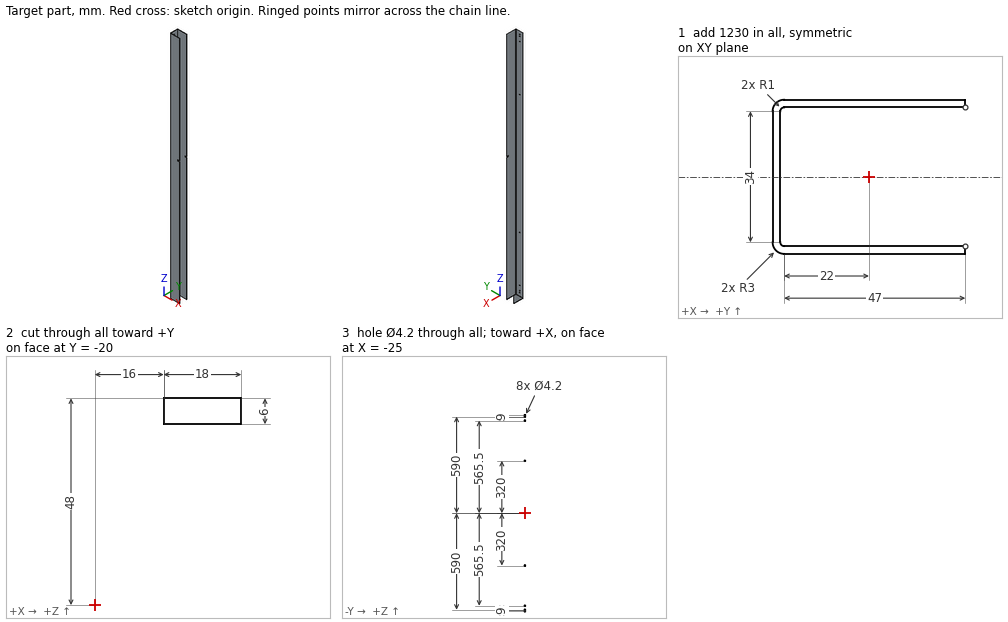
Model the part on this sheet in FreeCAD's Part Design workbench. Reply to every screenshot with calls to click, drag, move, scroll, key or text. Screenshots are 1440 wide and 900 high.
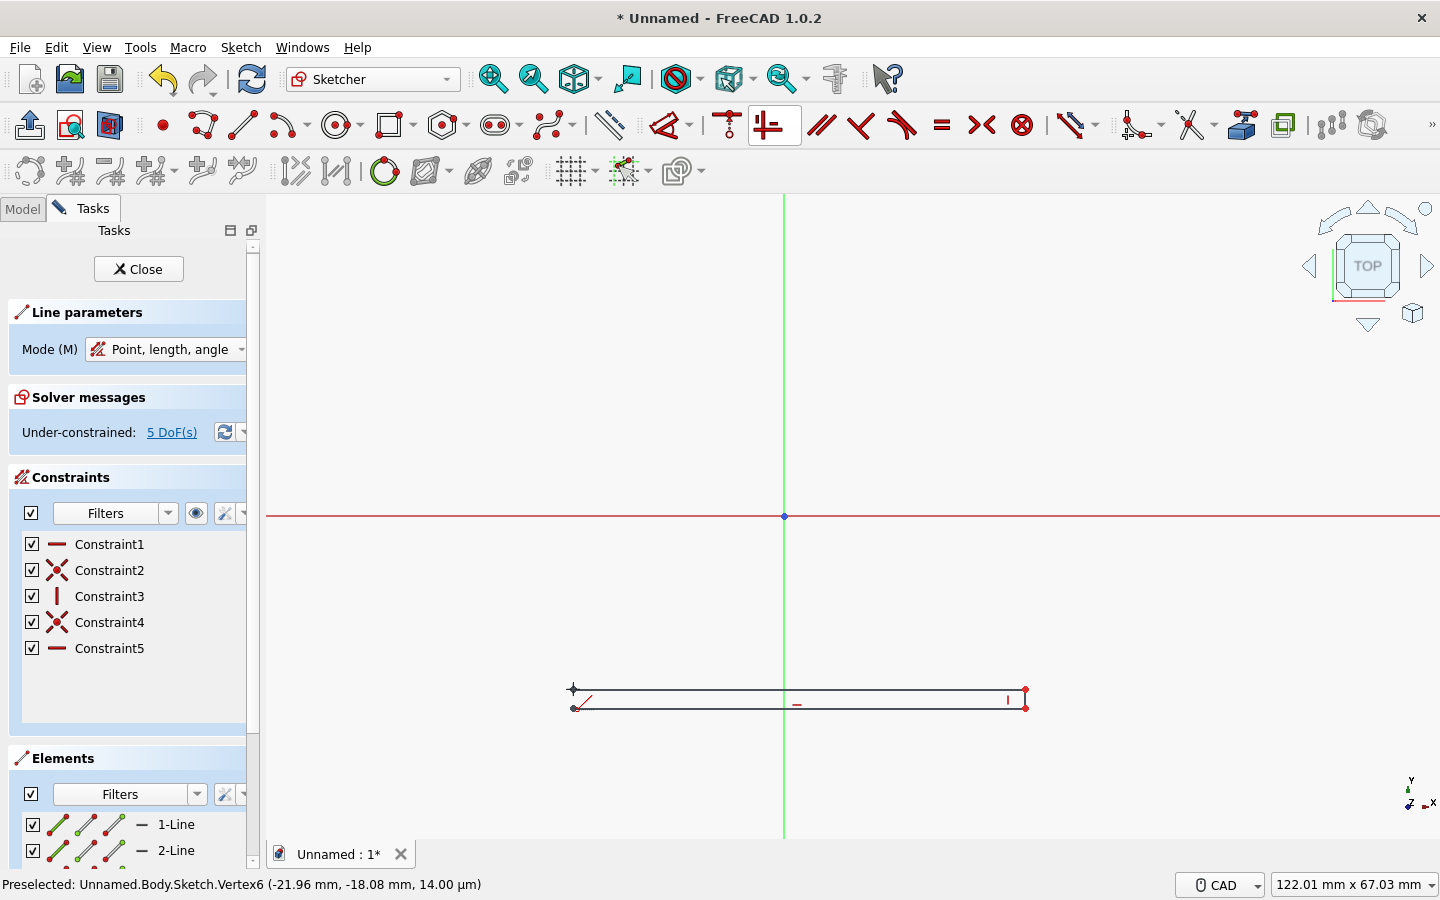
click(563, 680)
click(563, 352)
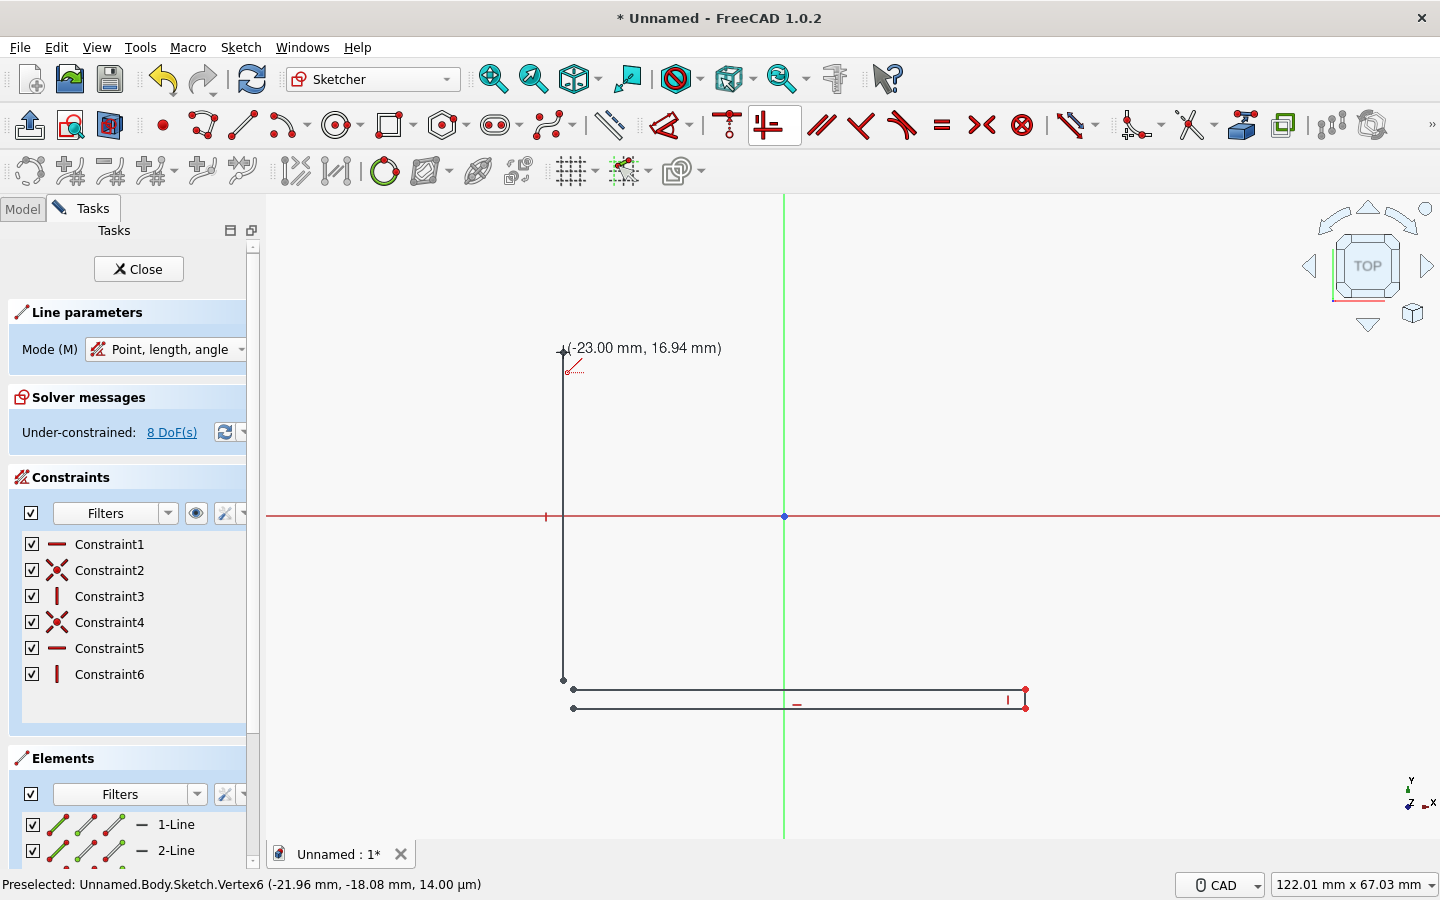
key(g)
key(m)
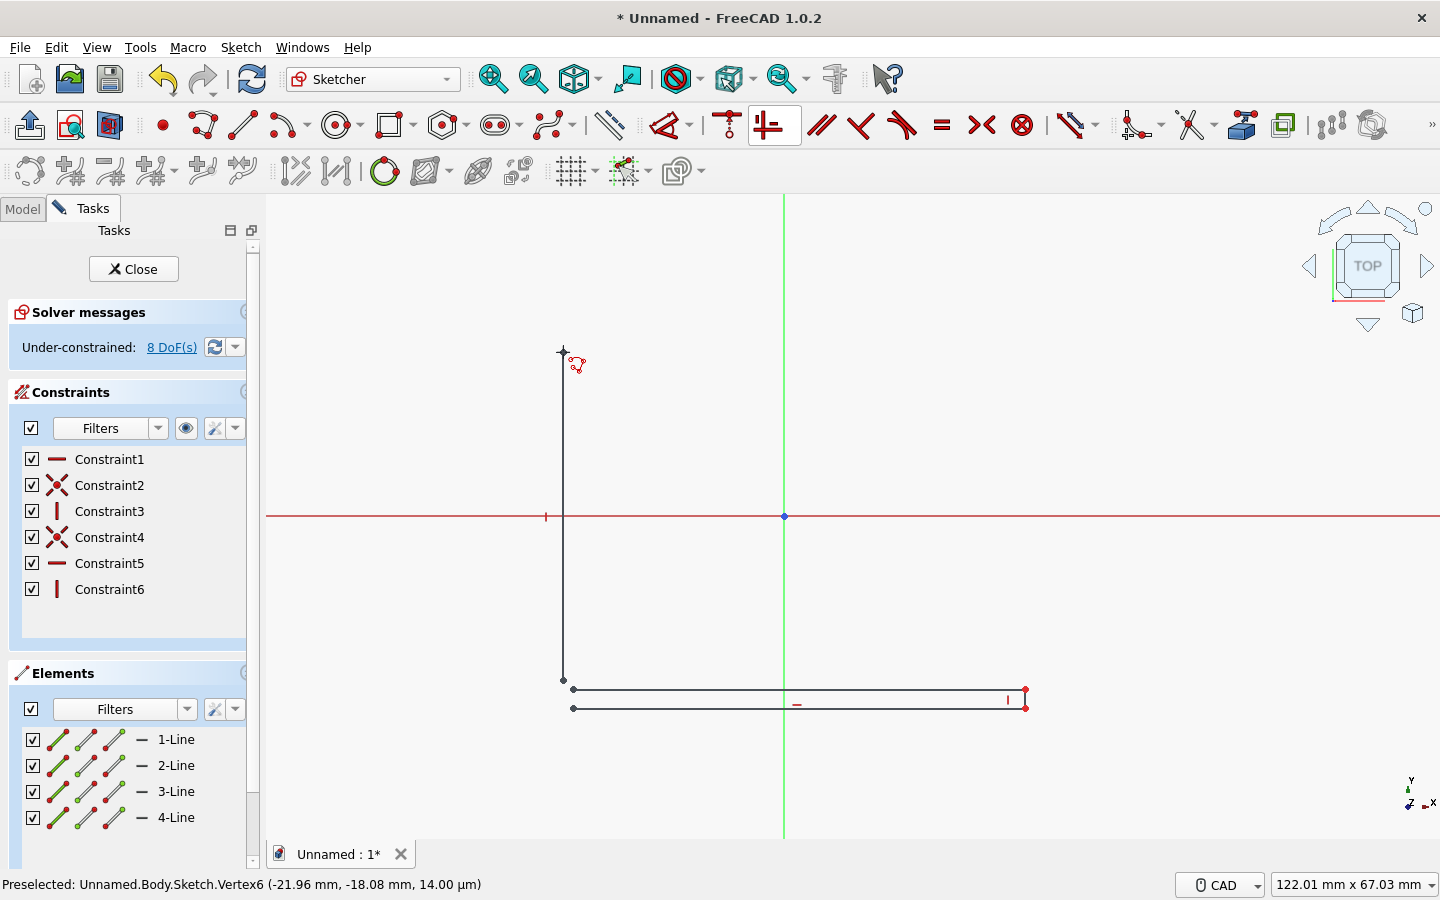
click(573, 343)
click(1025, 343)
click(1025, 324)
click(573, 324)
right_click(573, 324)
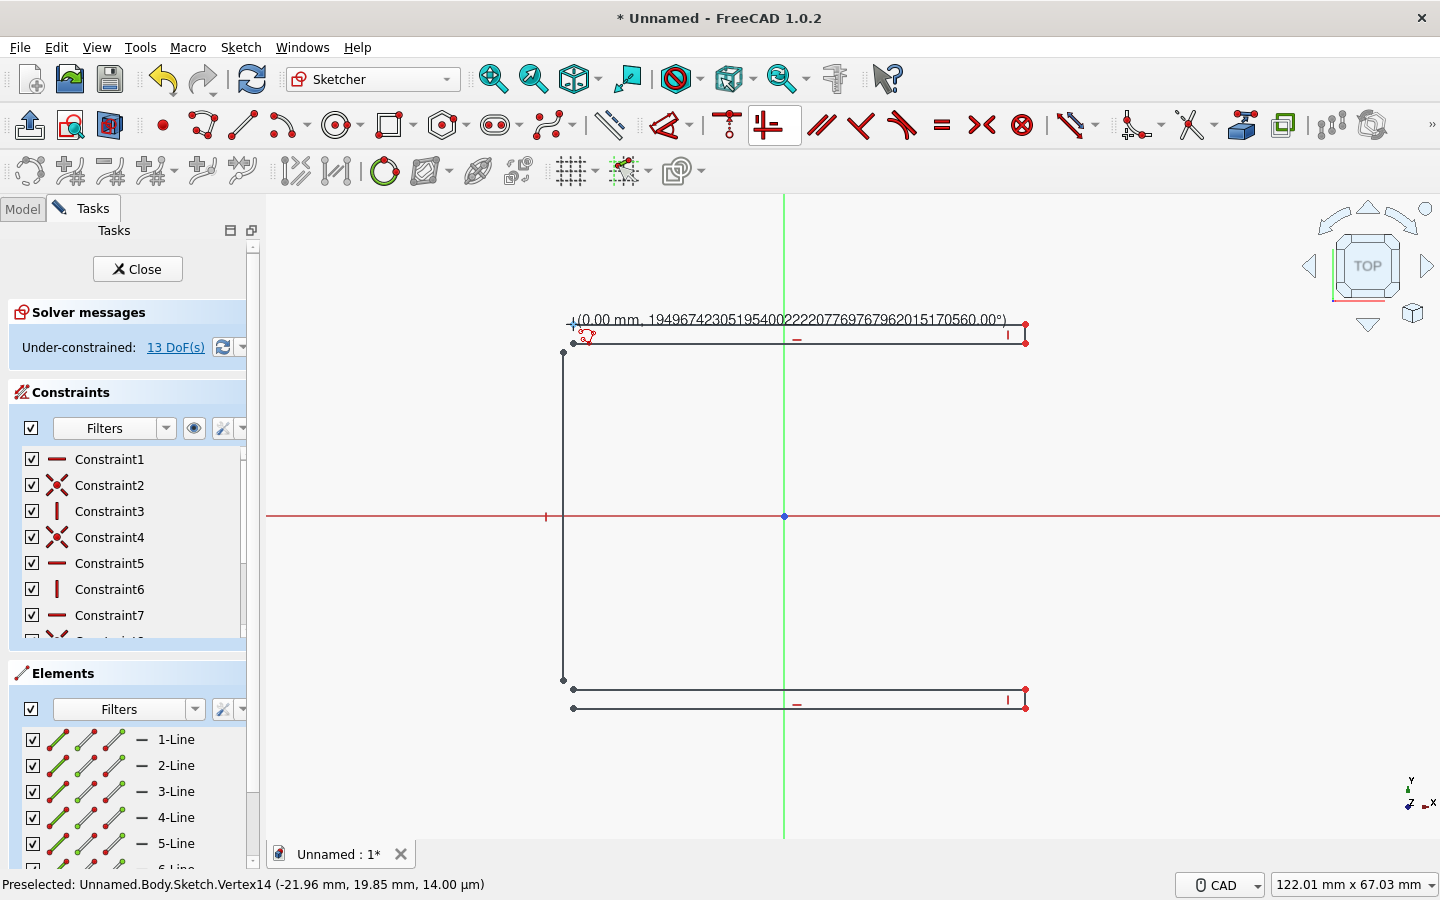
key(g)
key(l)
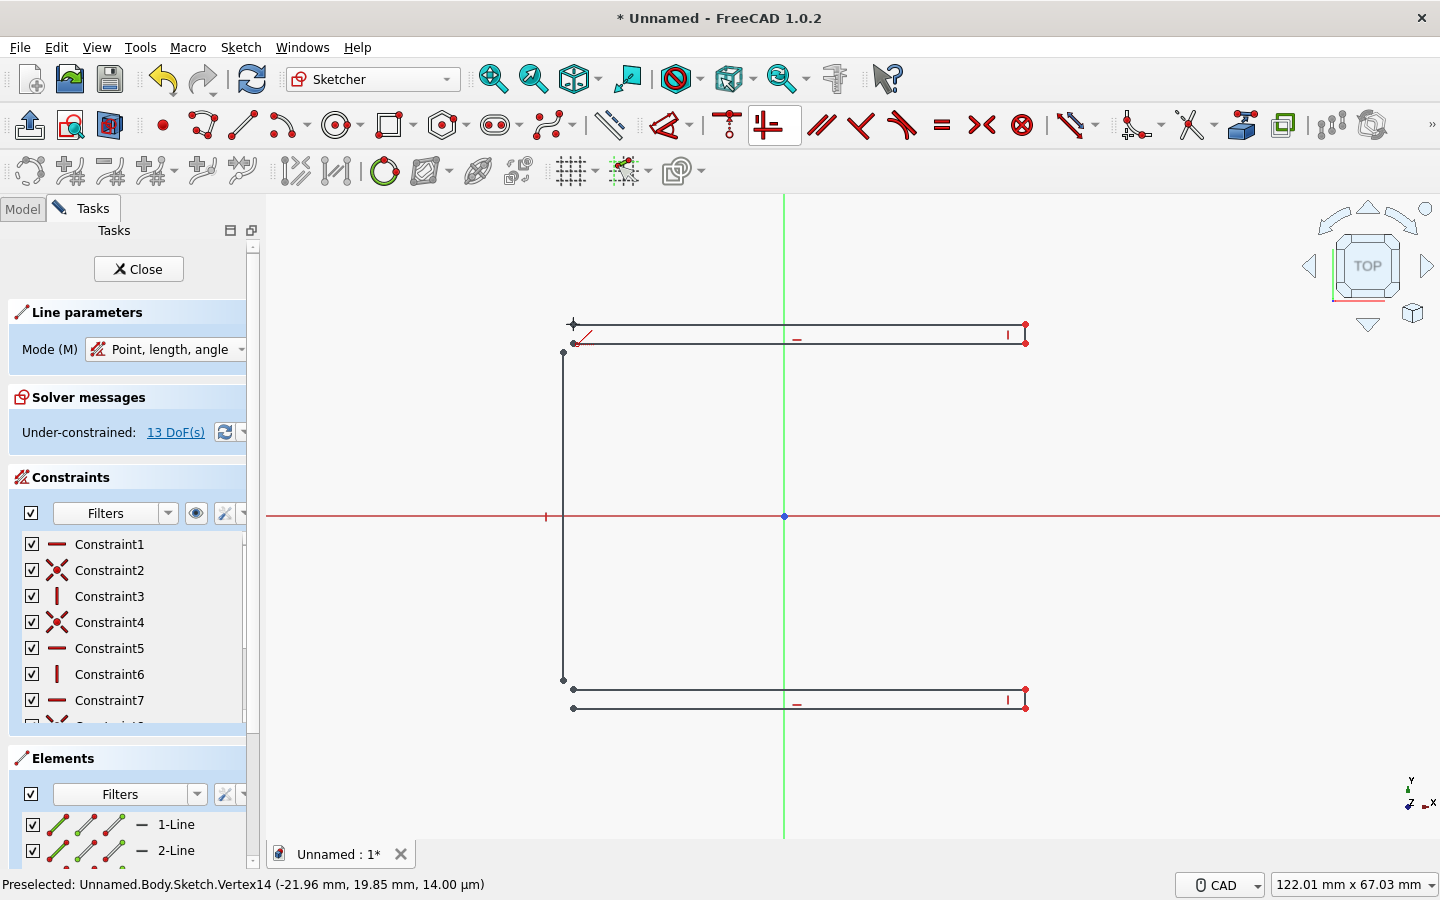
click(544, 352)
click(544, 680)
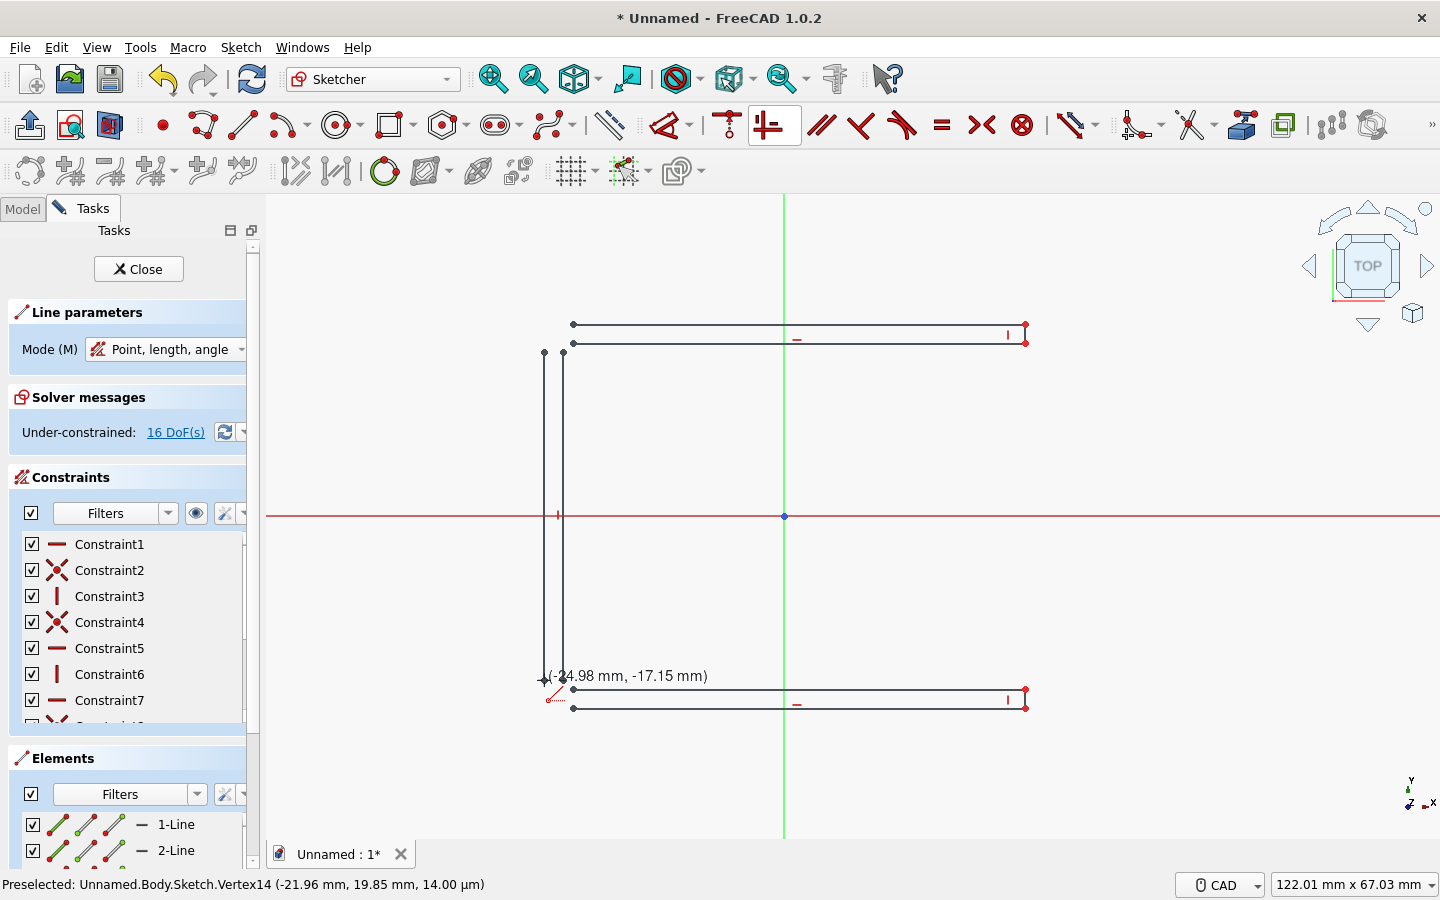
key(g)
key(3)
key(a)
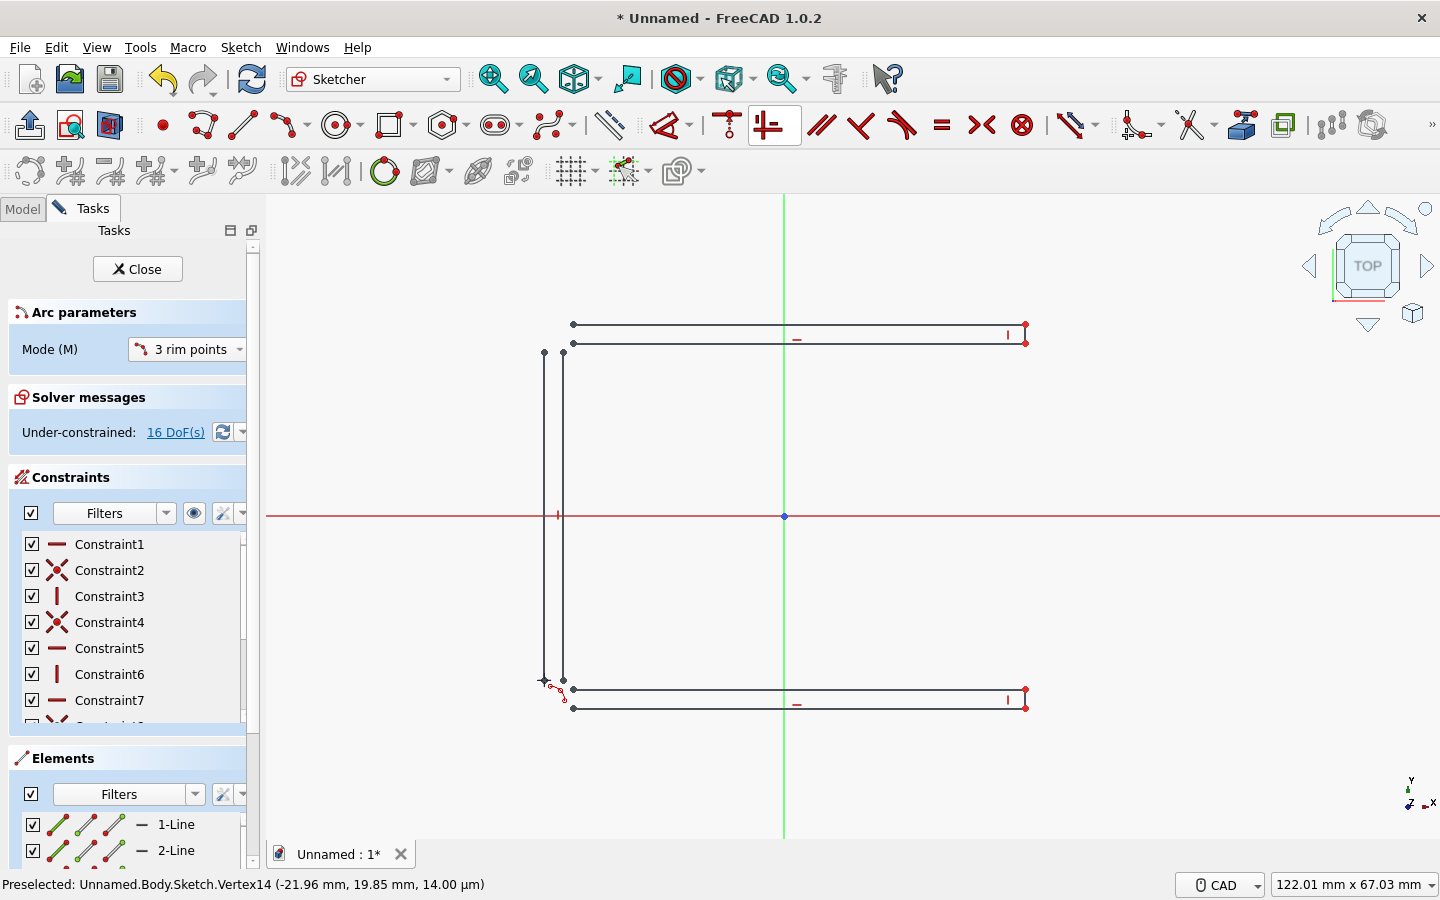
click(573, 690)
click(563, 681)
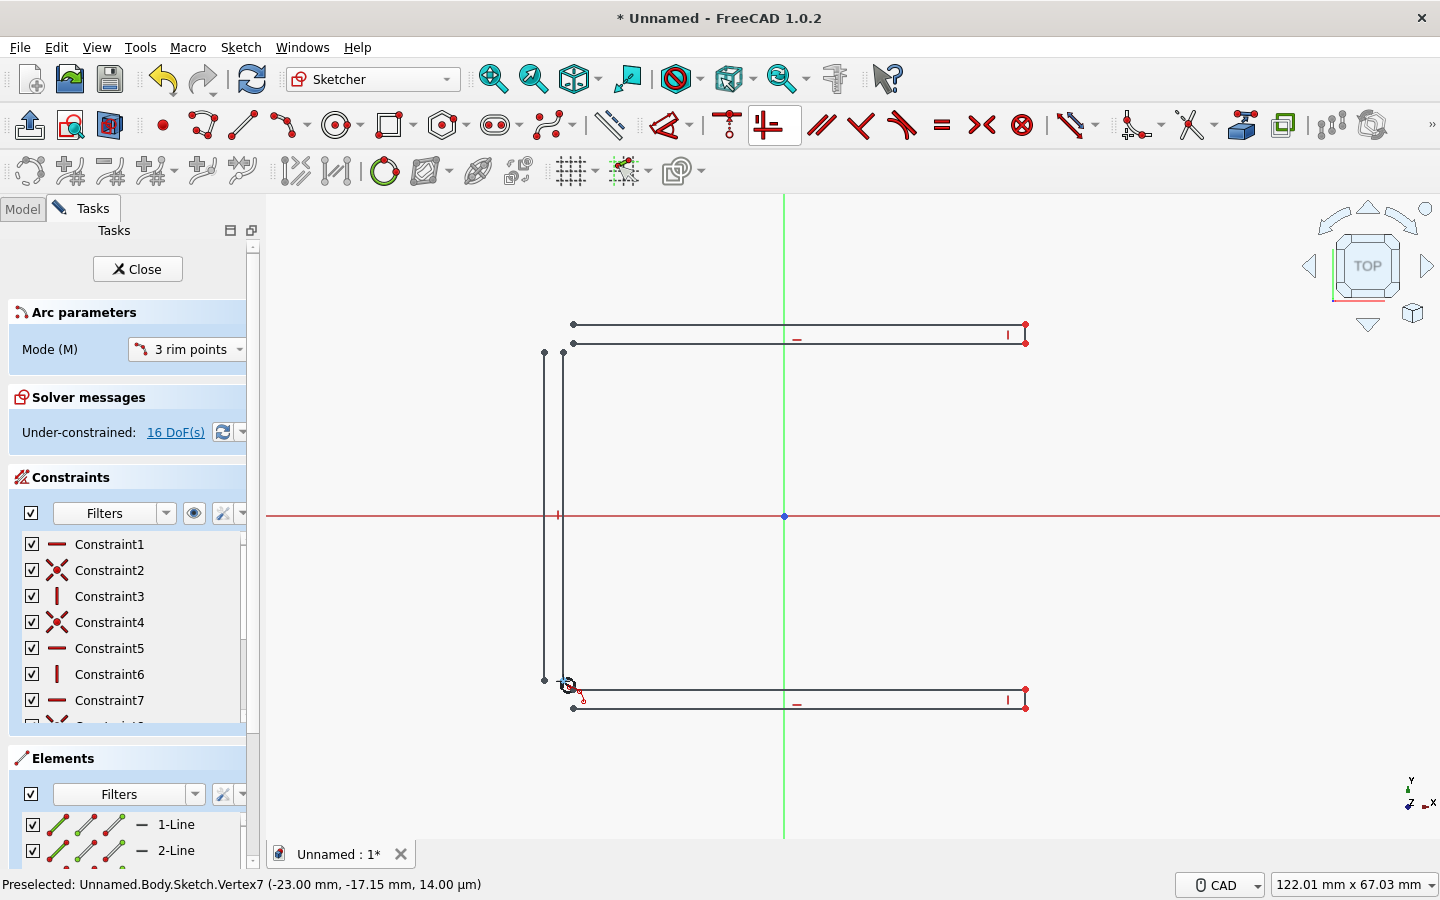
scroll(566, 686, up, 9)